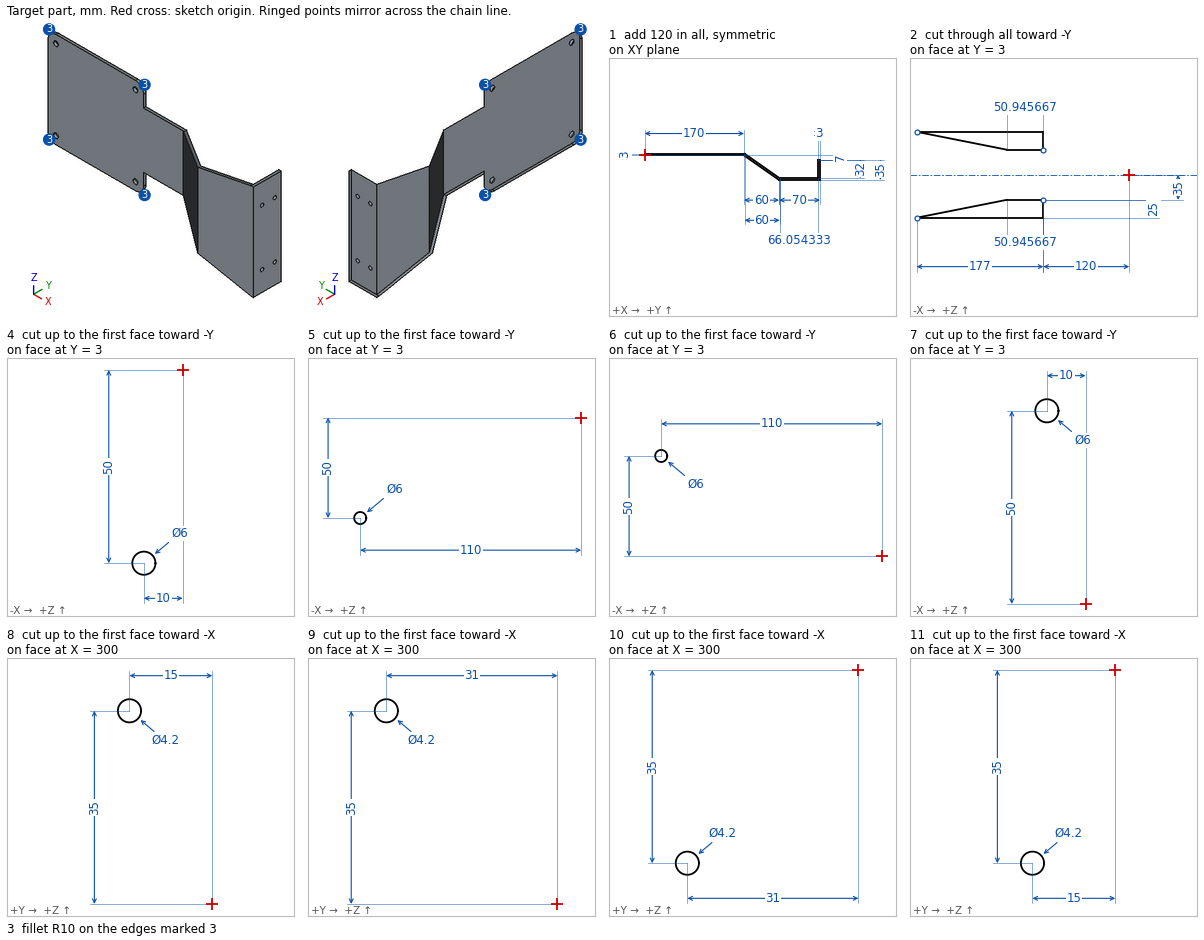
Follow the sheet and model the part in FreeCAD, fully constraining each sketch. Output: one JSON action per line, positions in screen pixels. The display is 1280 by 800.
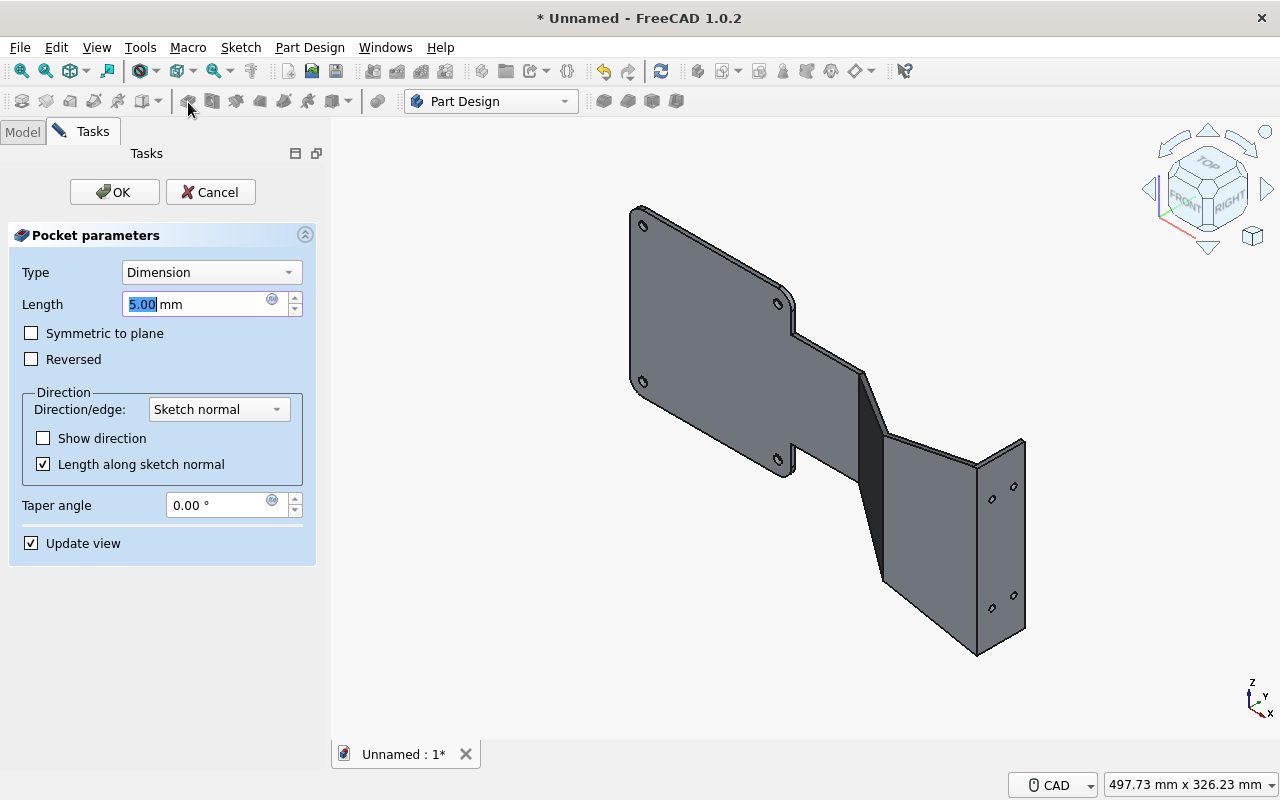
{"action": "left_click", "coordinate": [212, 272]}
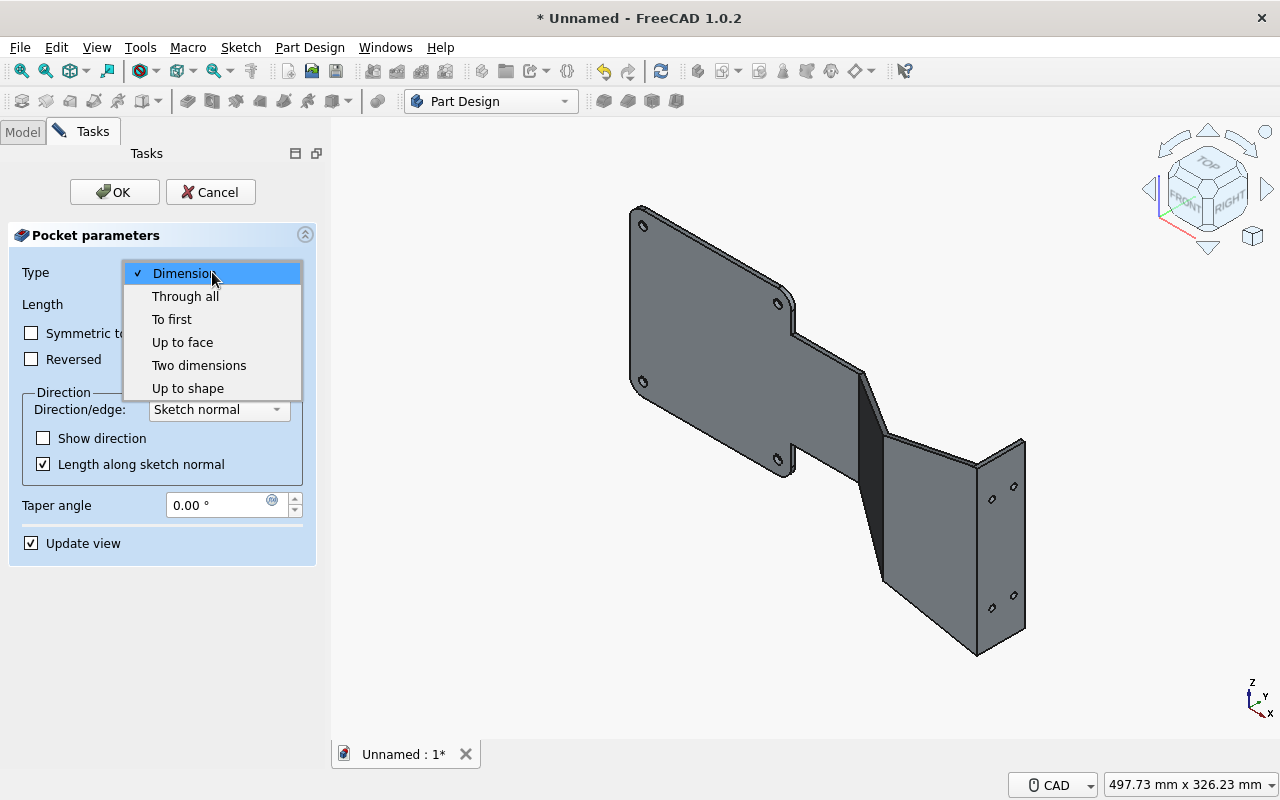
{"action": "left_click", "coordinate": [212, 320]}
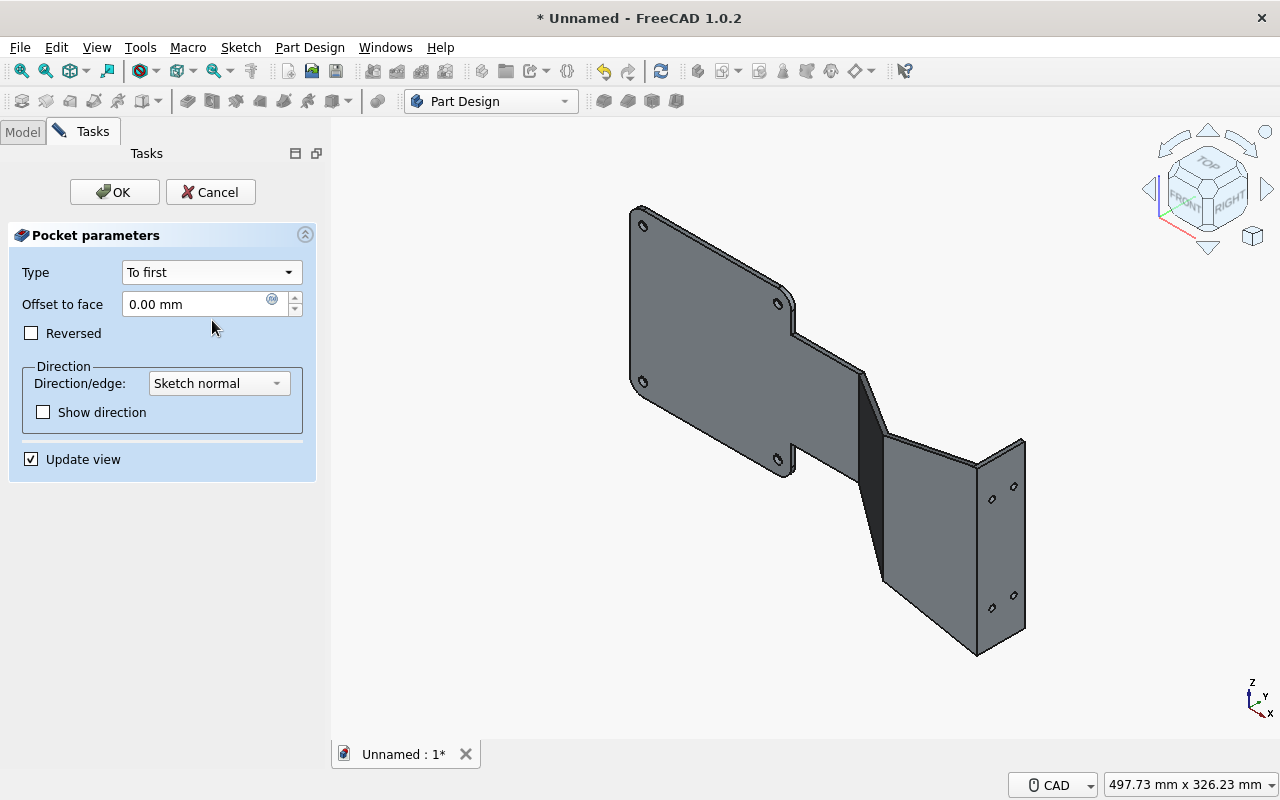
{"action": "left_click", "coordinate": [115, 192]}